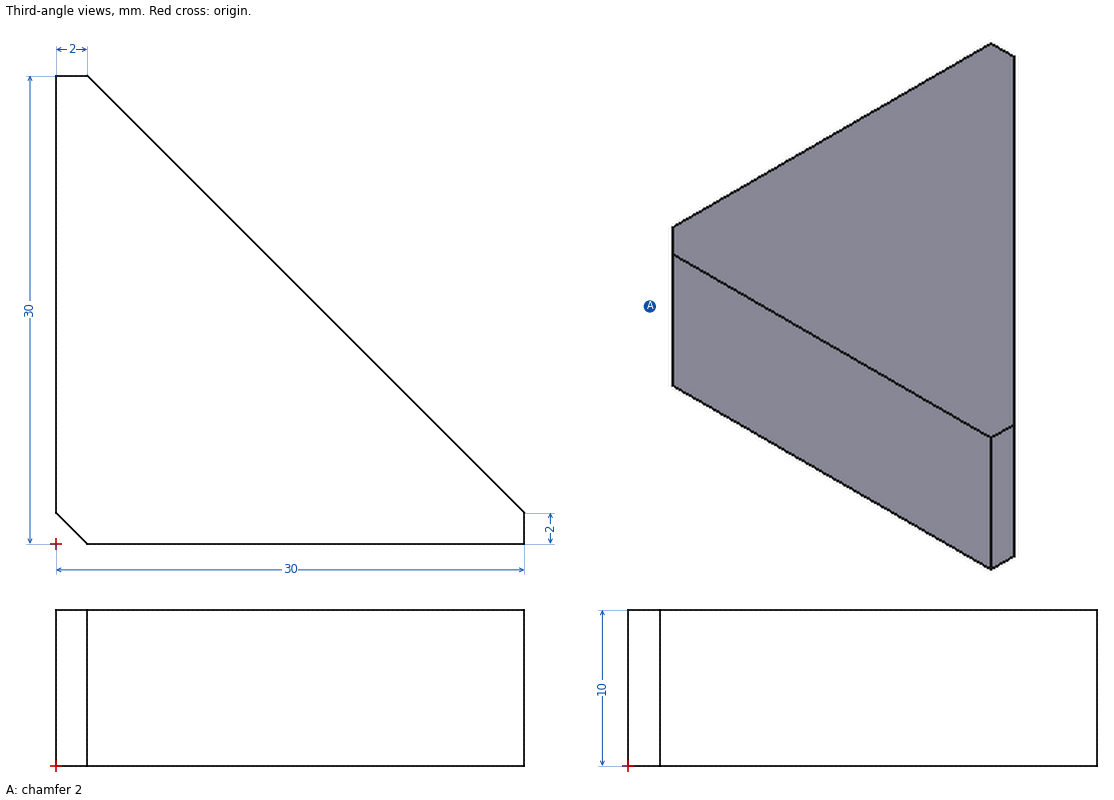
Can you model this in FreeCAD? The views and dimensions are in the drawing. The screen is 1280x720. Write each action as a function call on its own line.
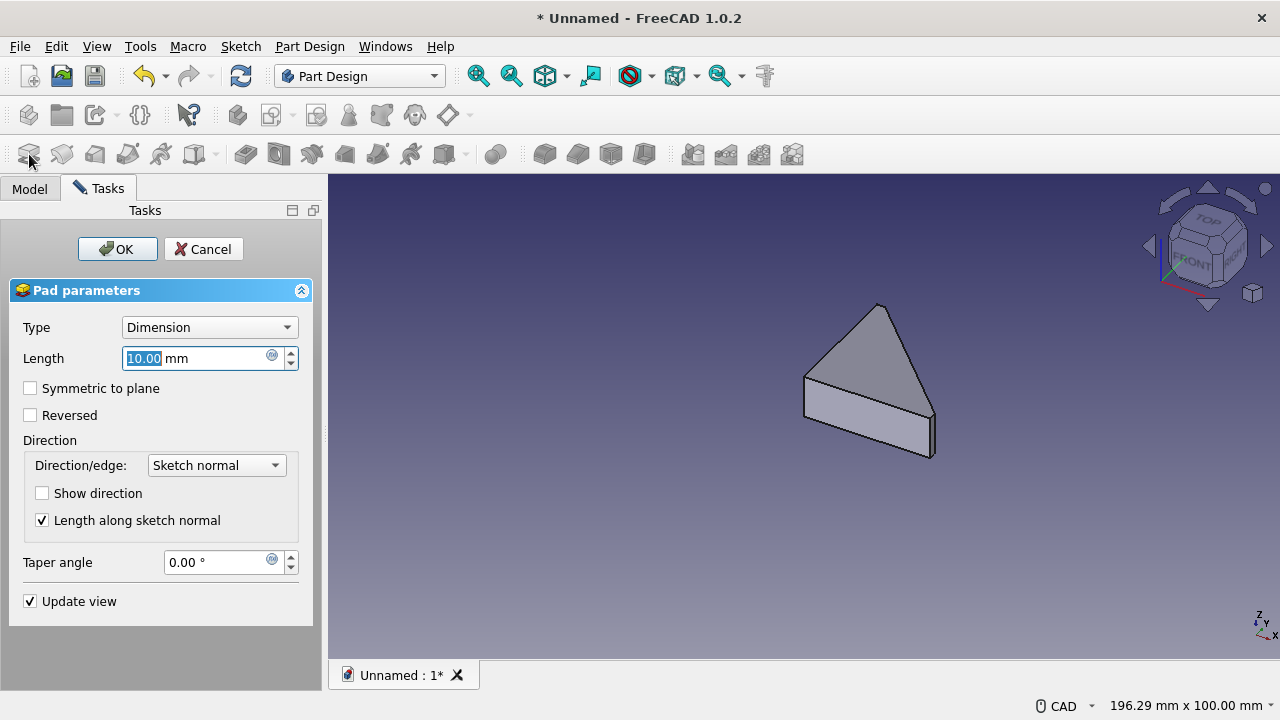
text(10)
key(Tab)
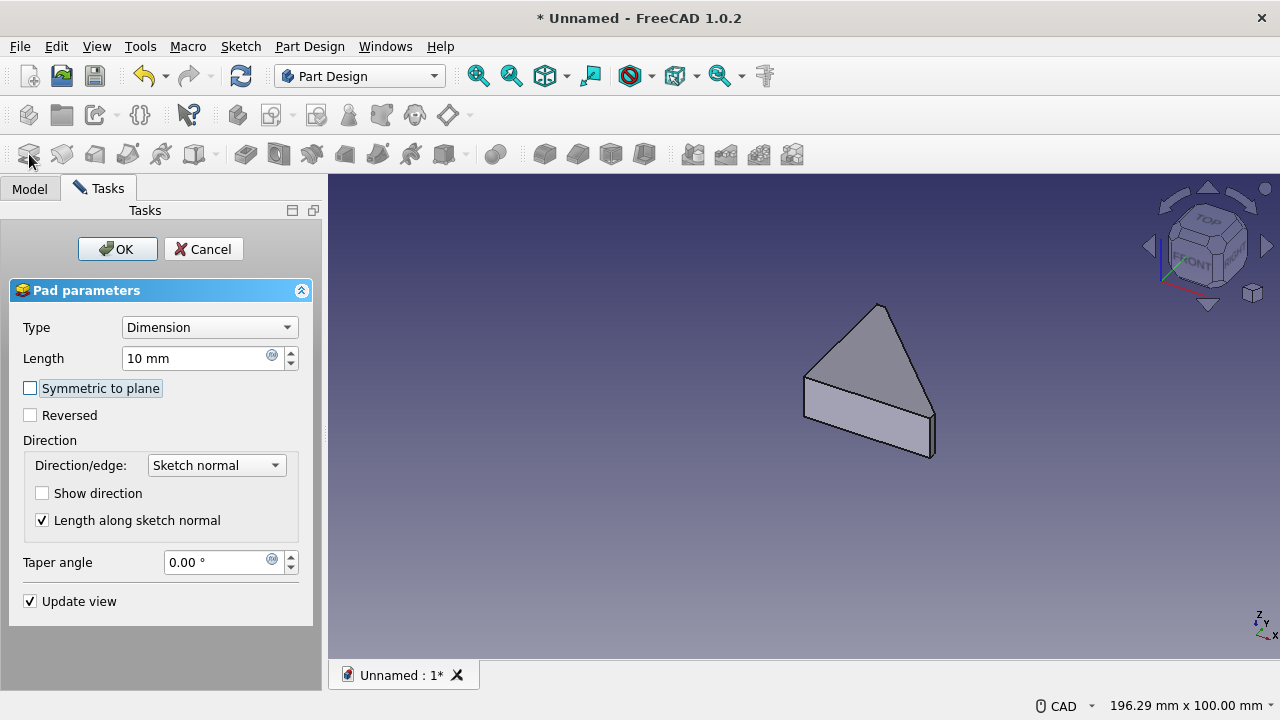
click(118, 249)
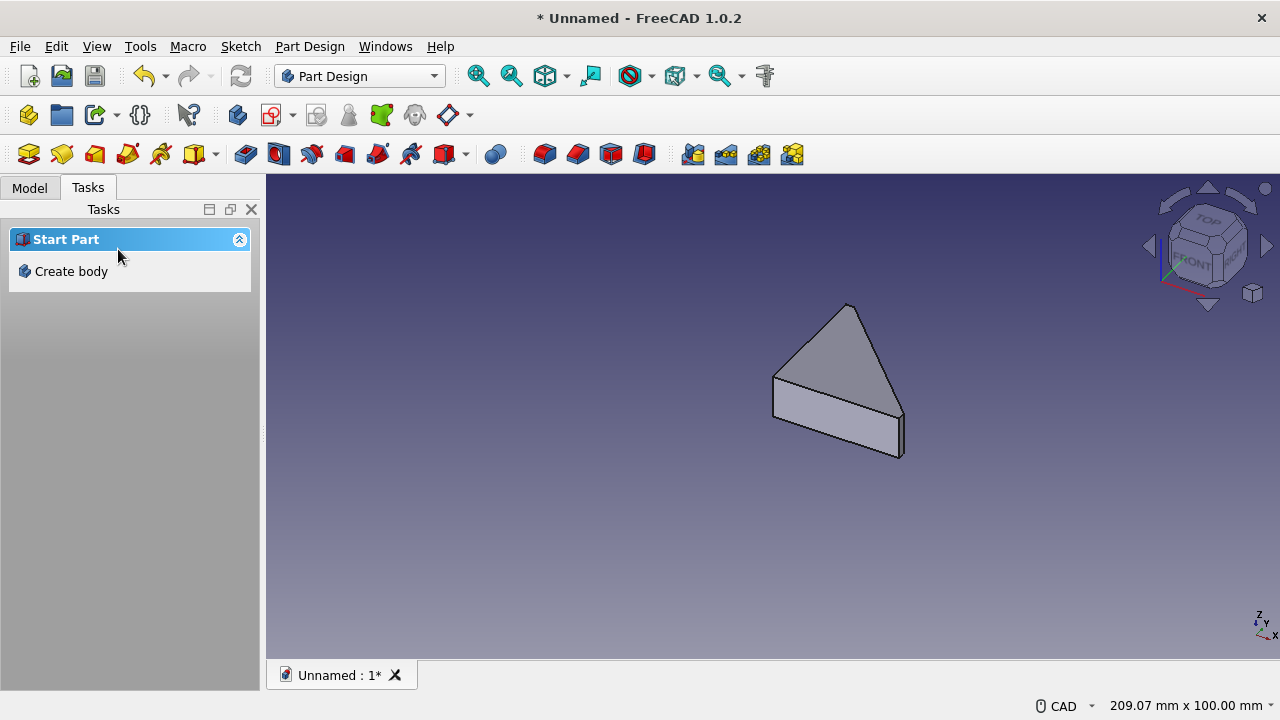
click(479, 76)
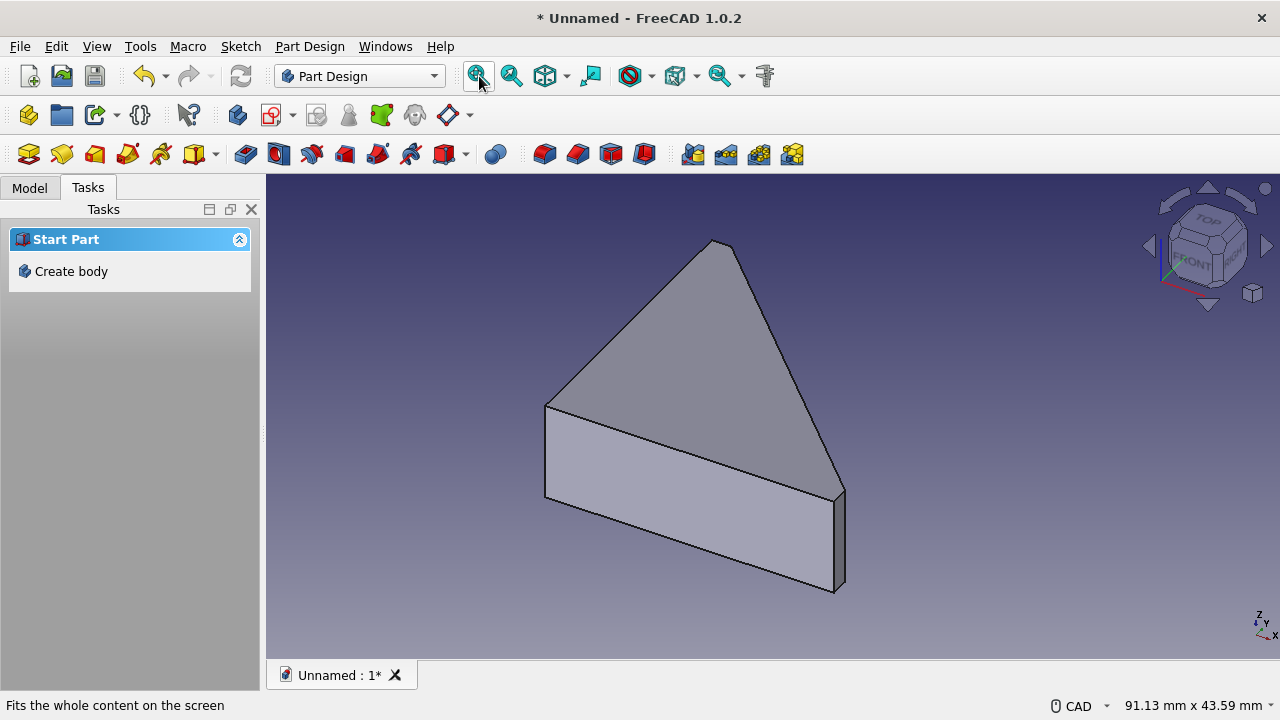
key(0)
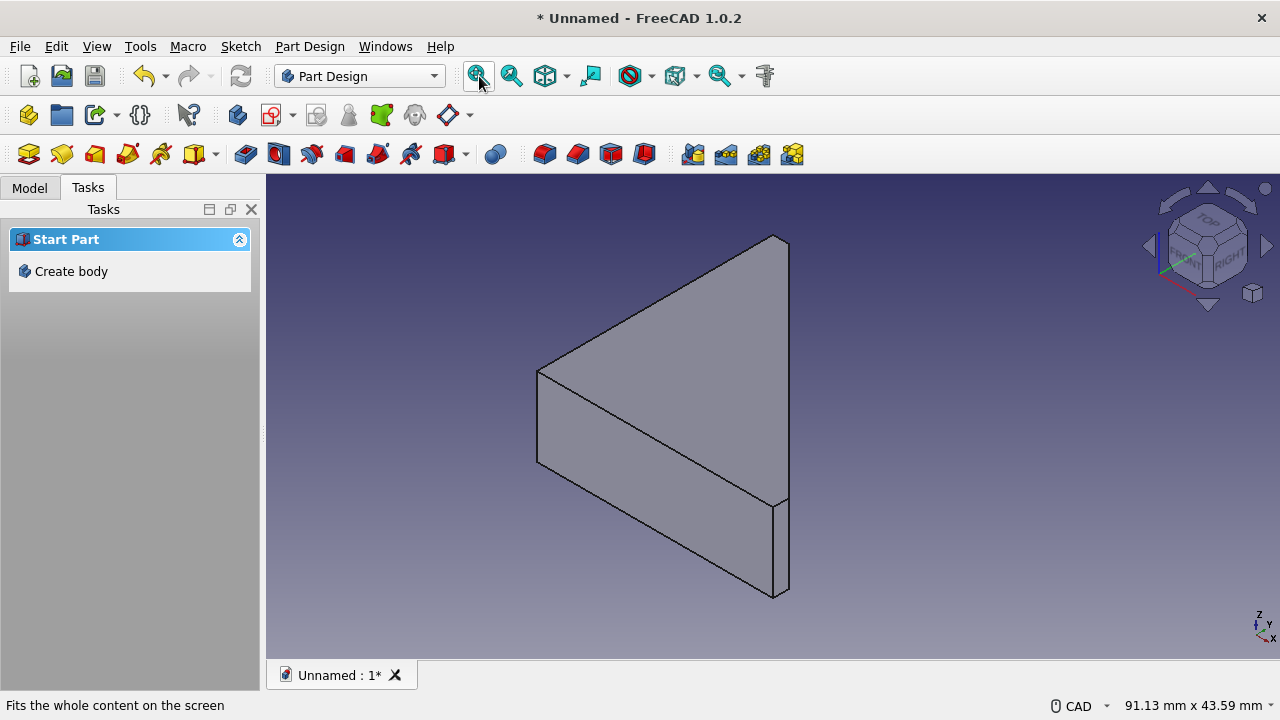
key(2)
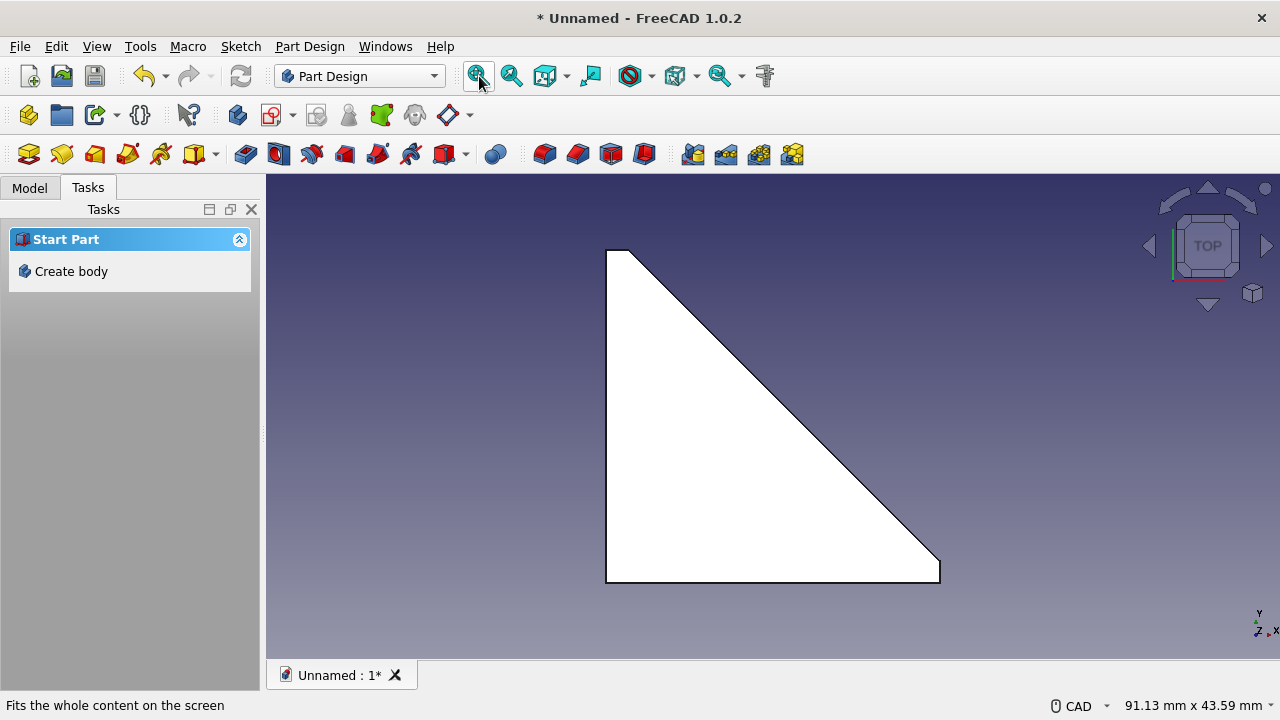
key(1)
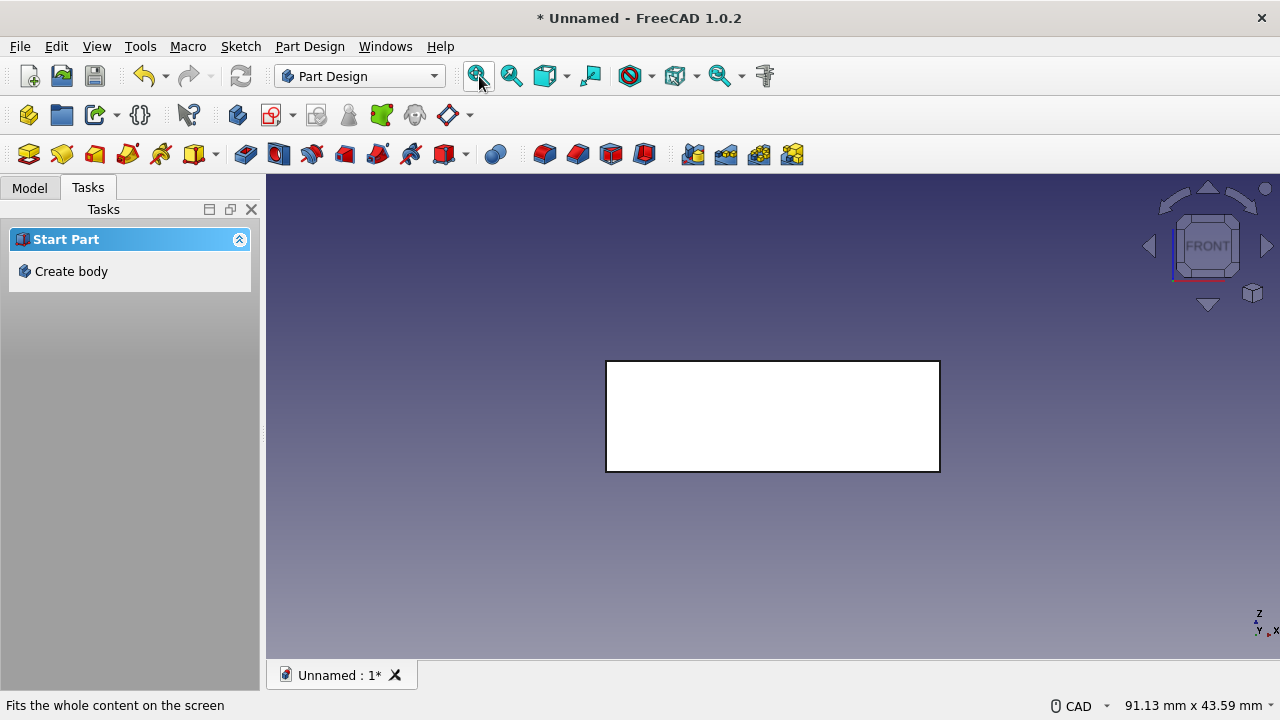
click(479, 76)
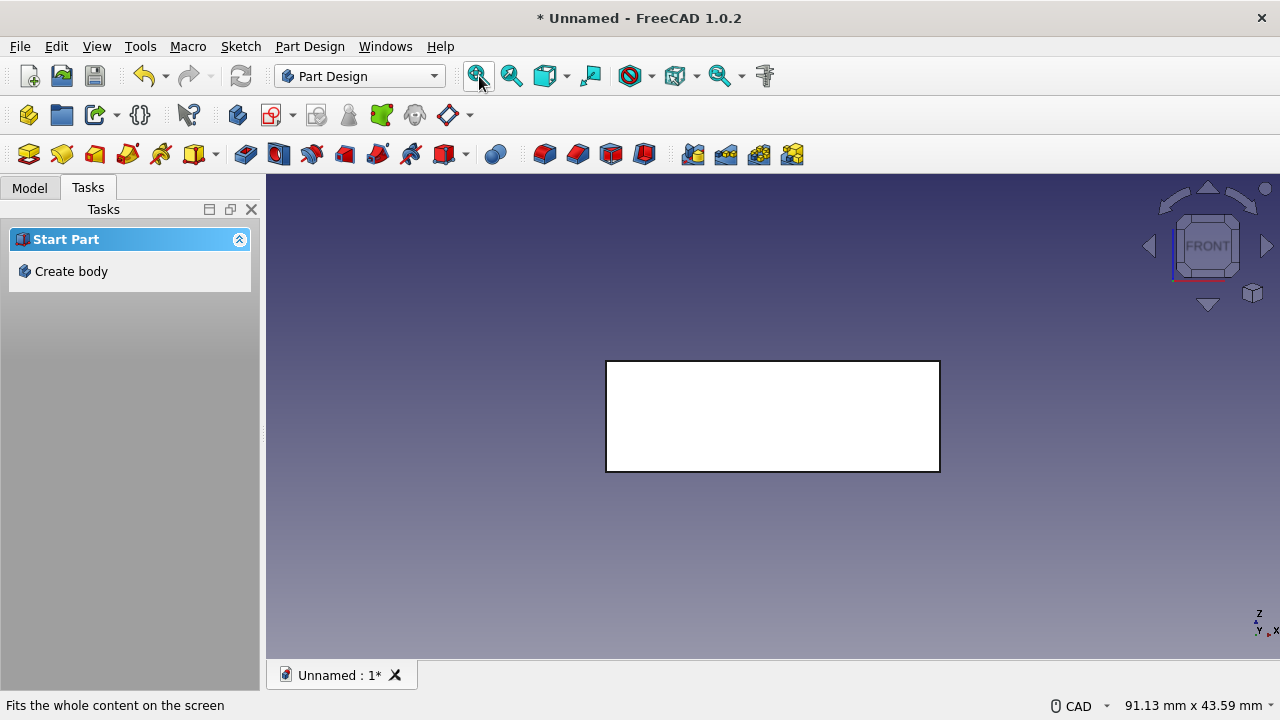
click(606, 416)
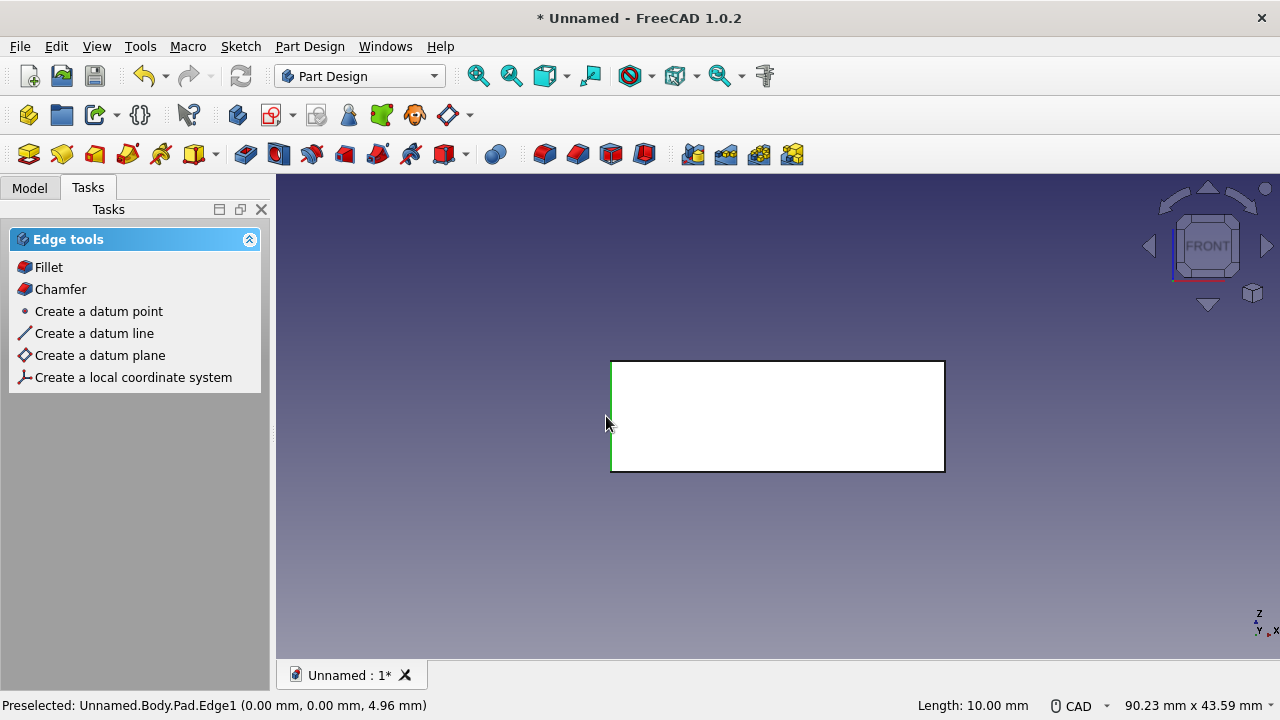
click(578, 154)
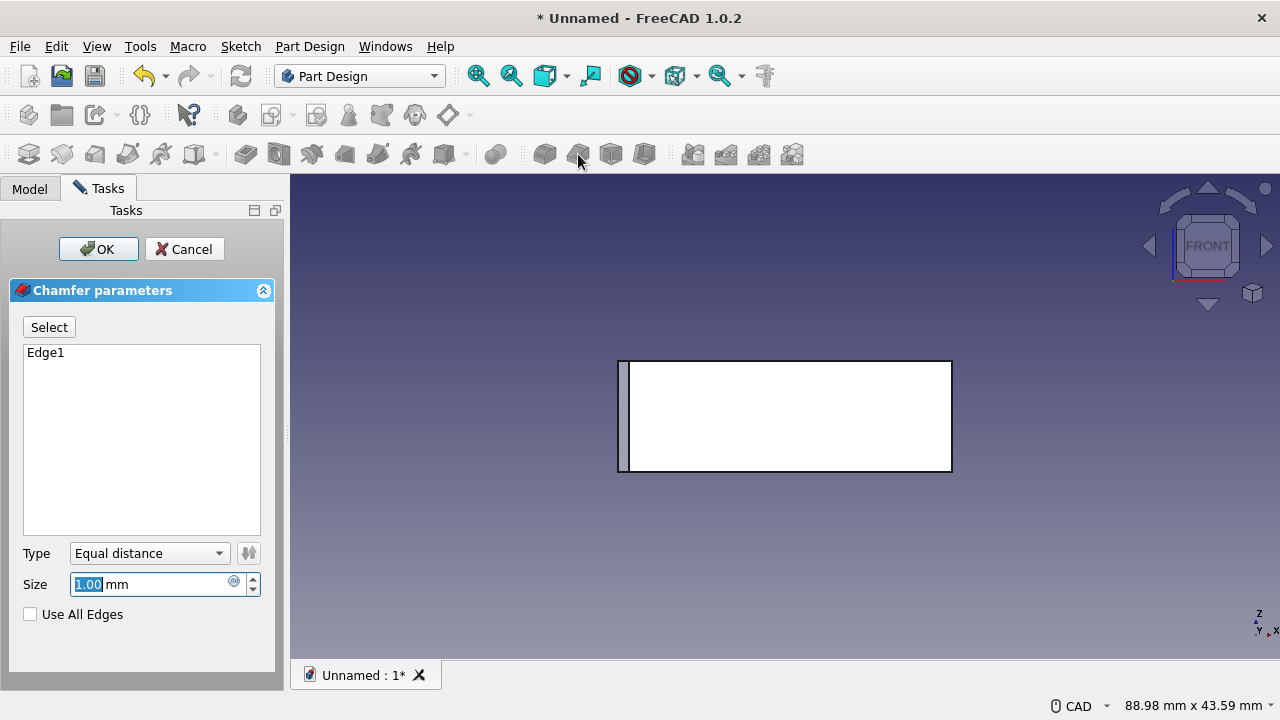
text(2)
key(Tab)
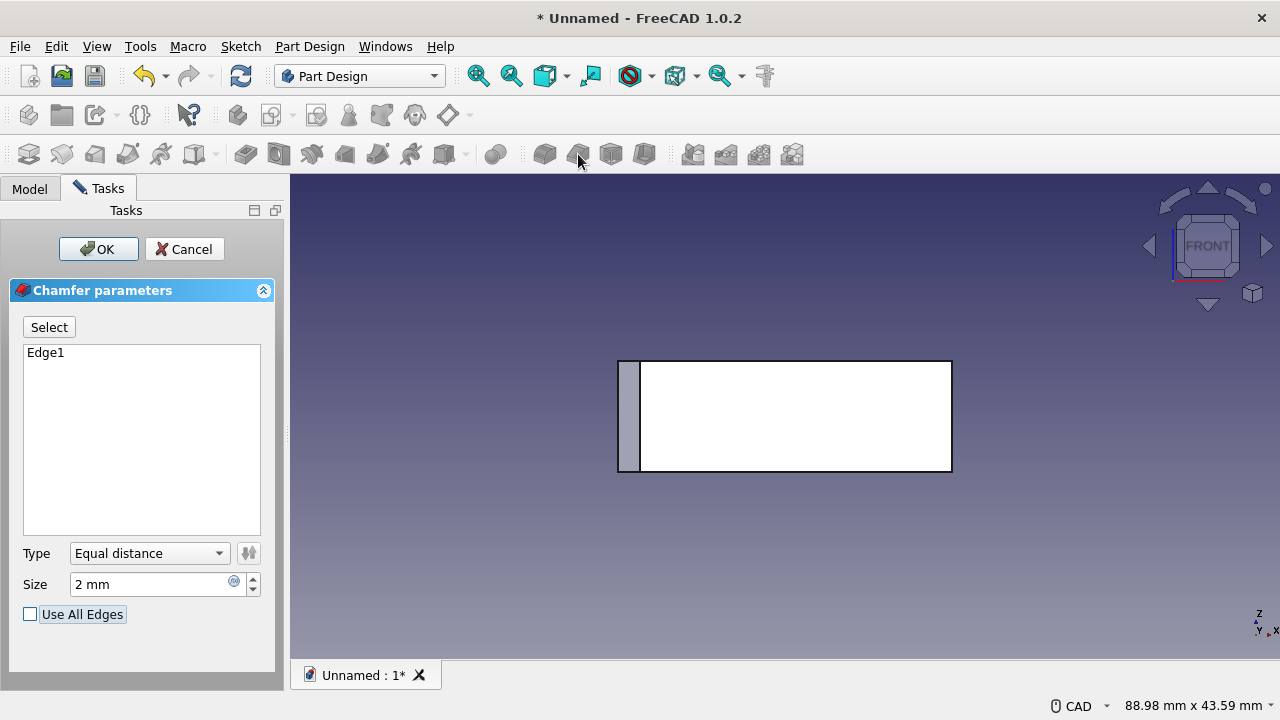
click(99, 249)